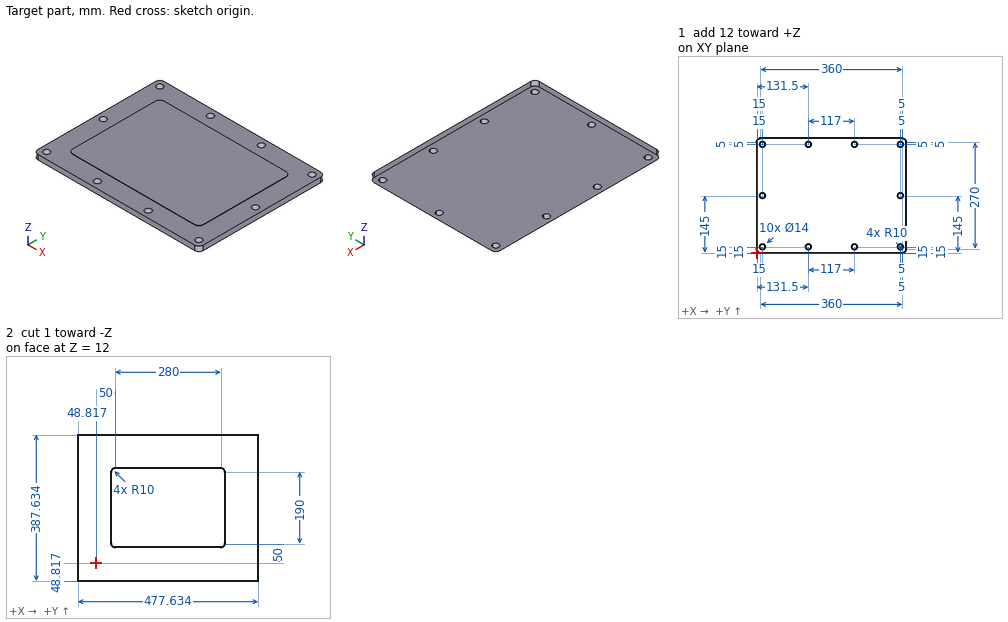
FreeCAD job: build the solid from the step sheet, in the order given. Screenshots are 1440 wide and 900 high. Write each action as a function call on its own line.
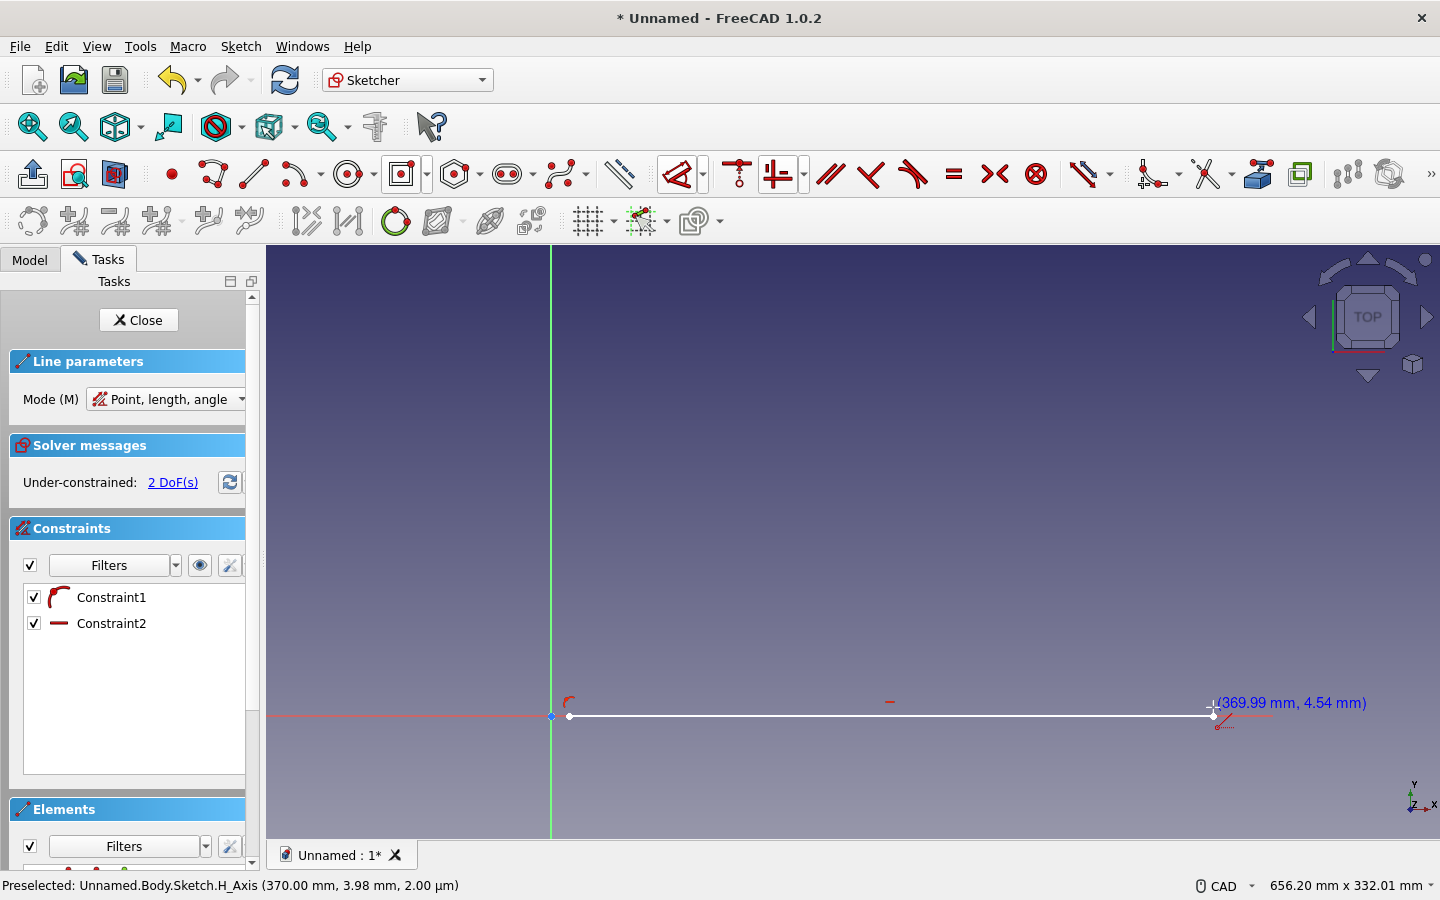
click(1231, 698)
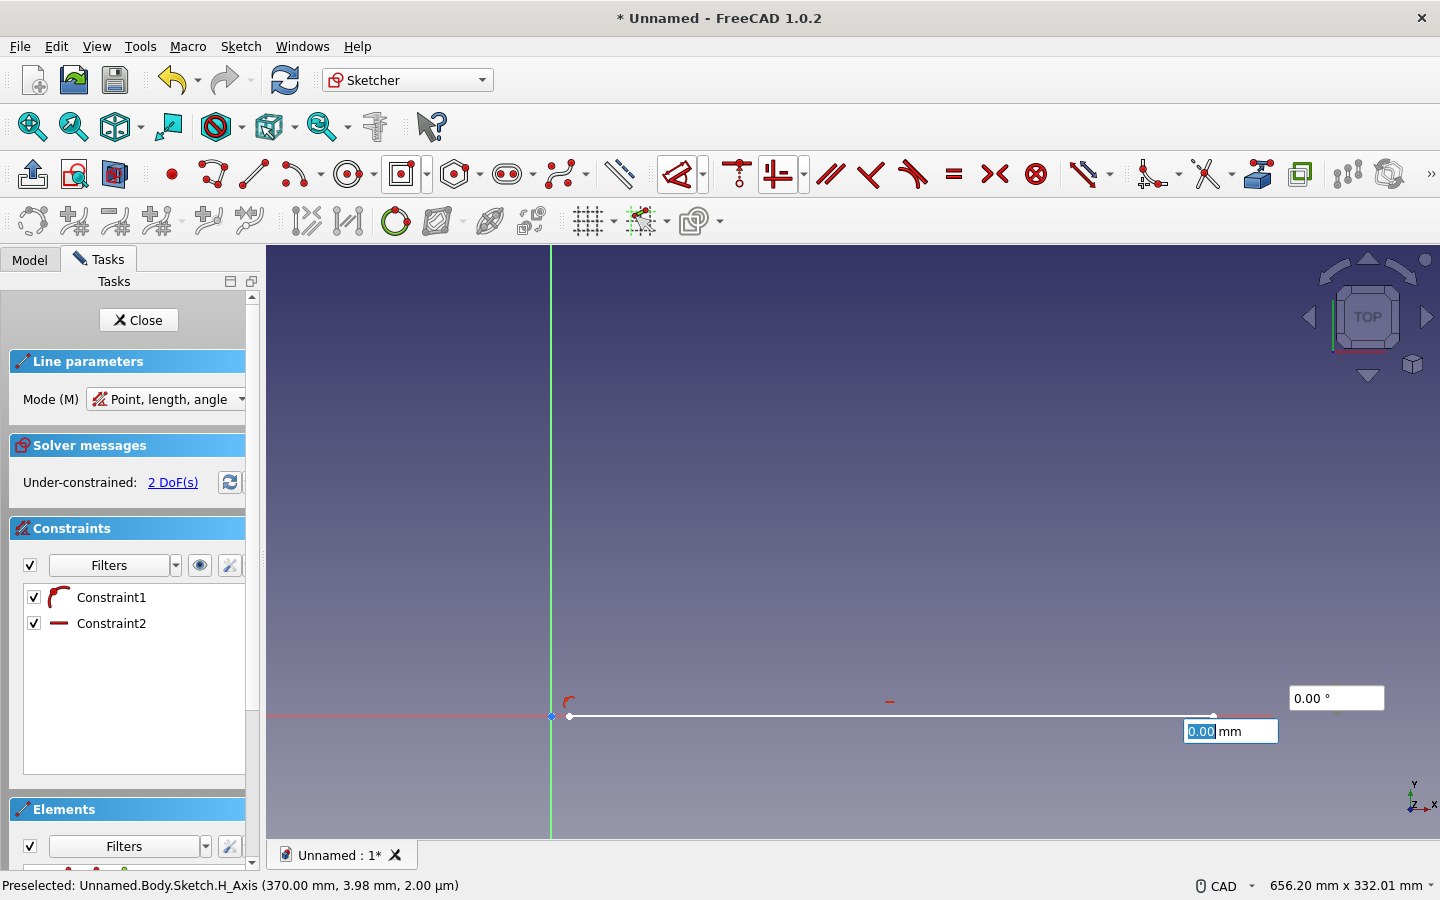
scroll(568, 715, down, 2)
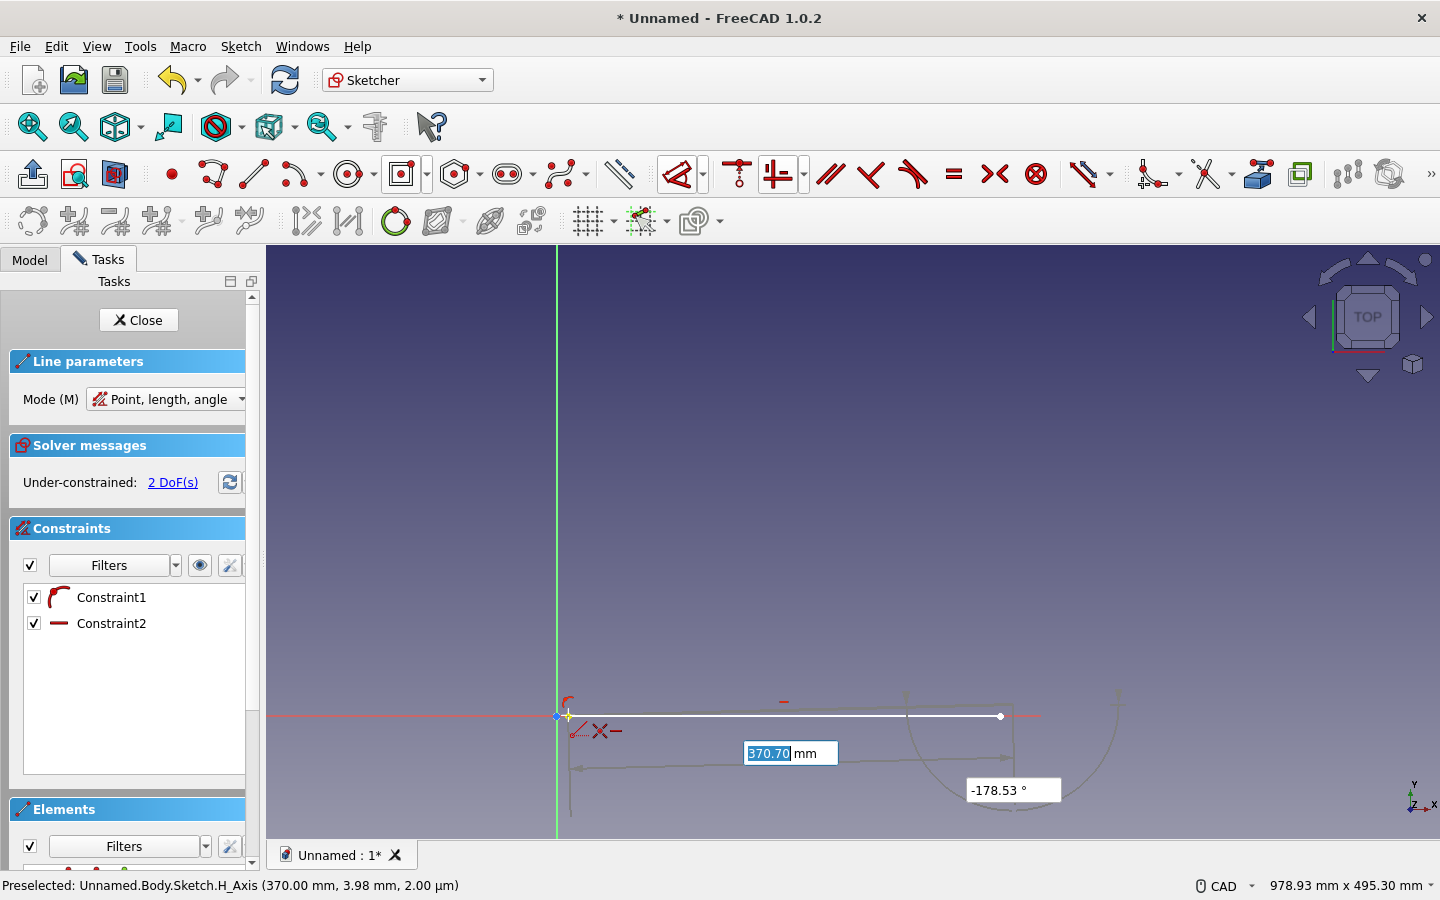
click(1013, 380)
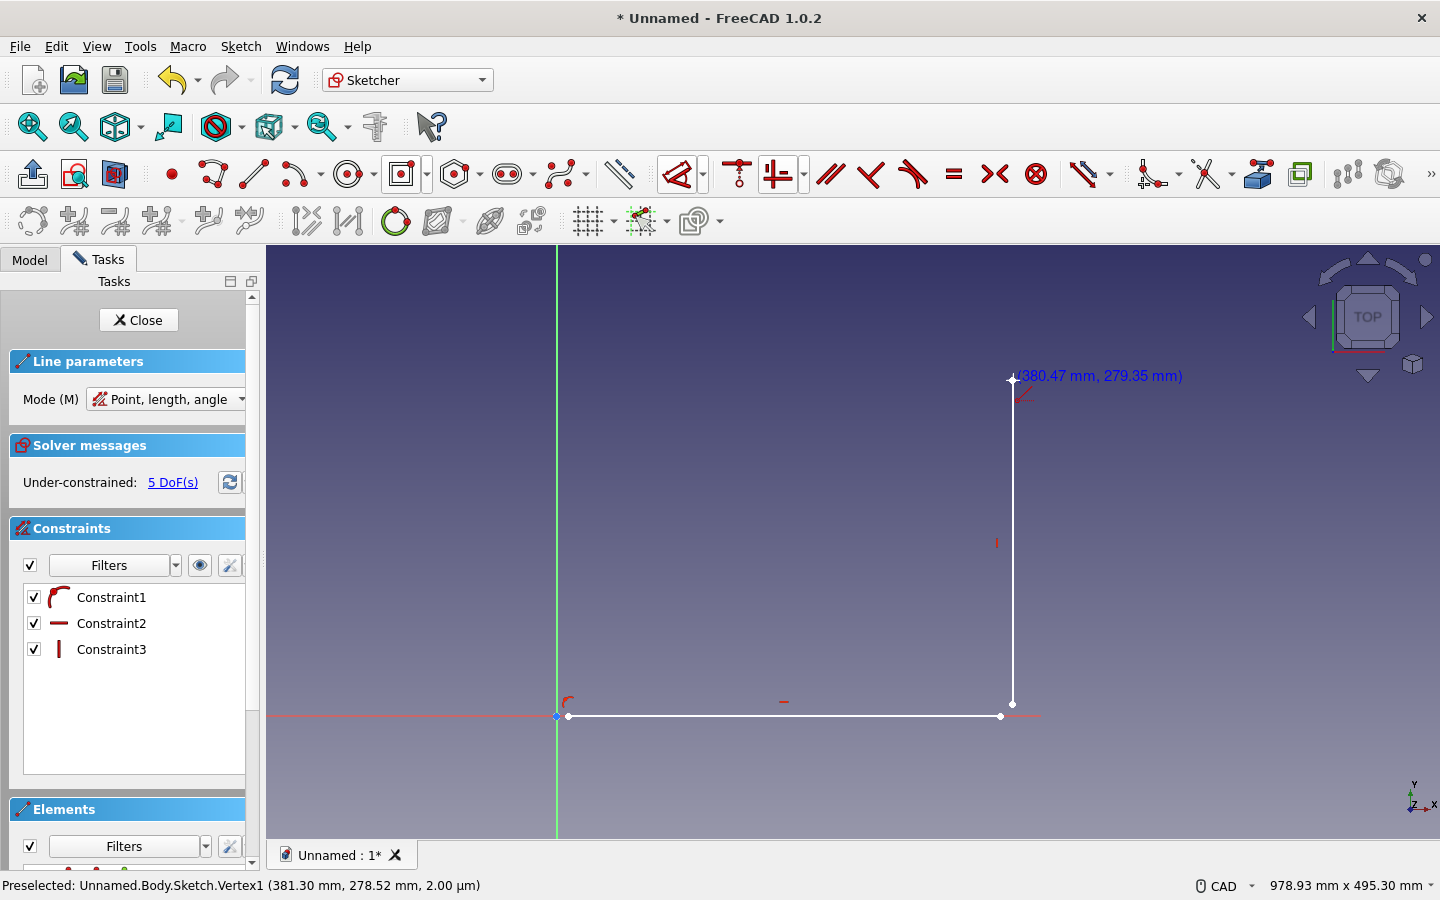
click(1000, 368)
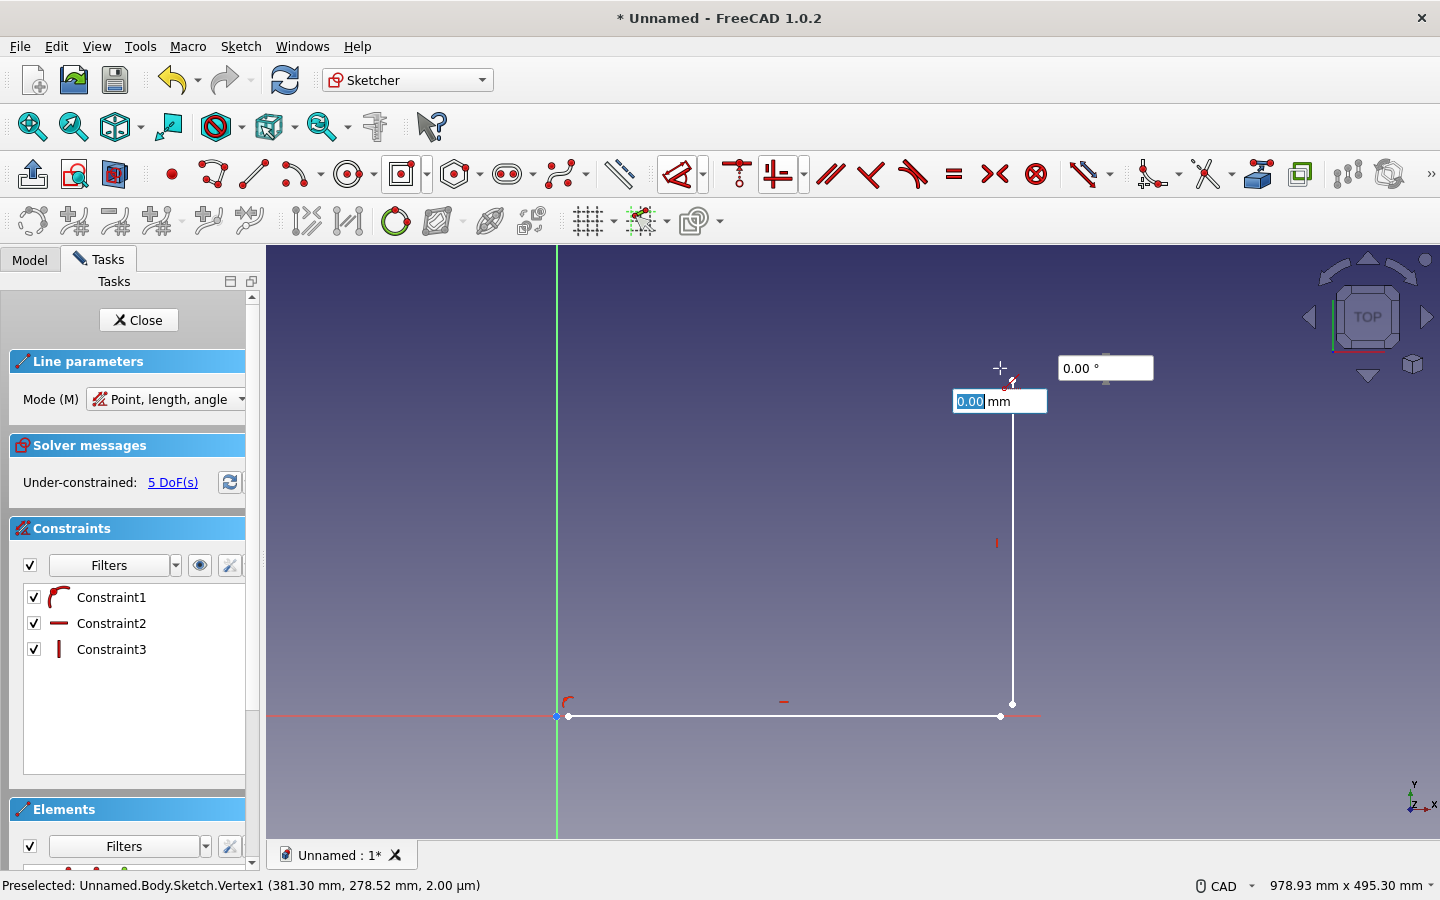
scroll(569, 368, up, 2)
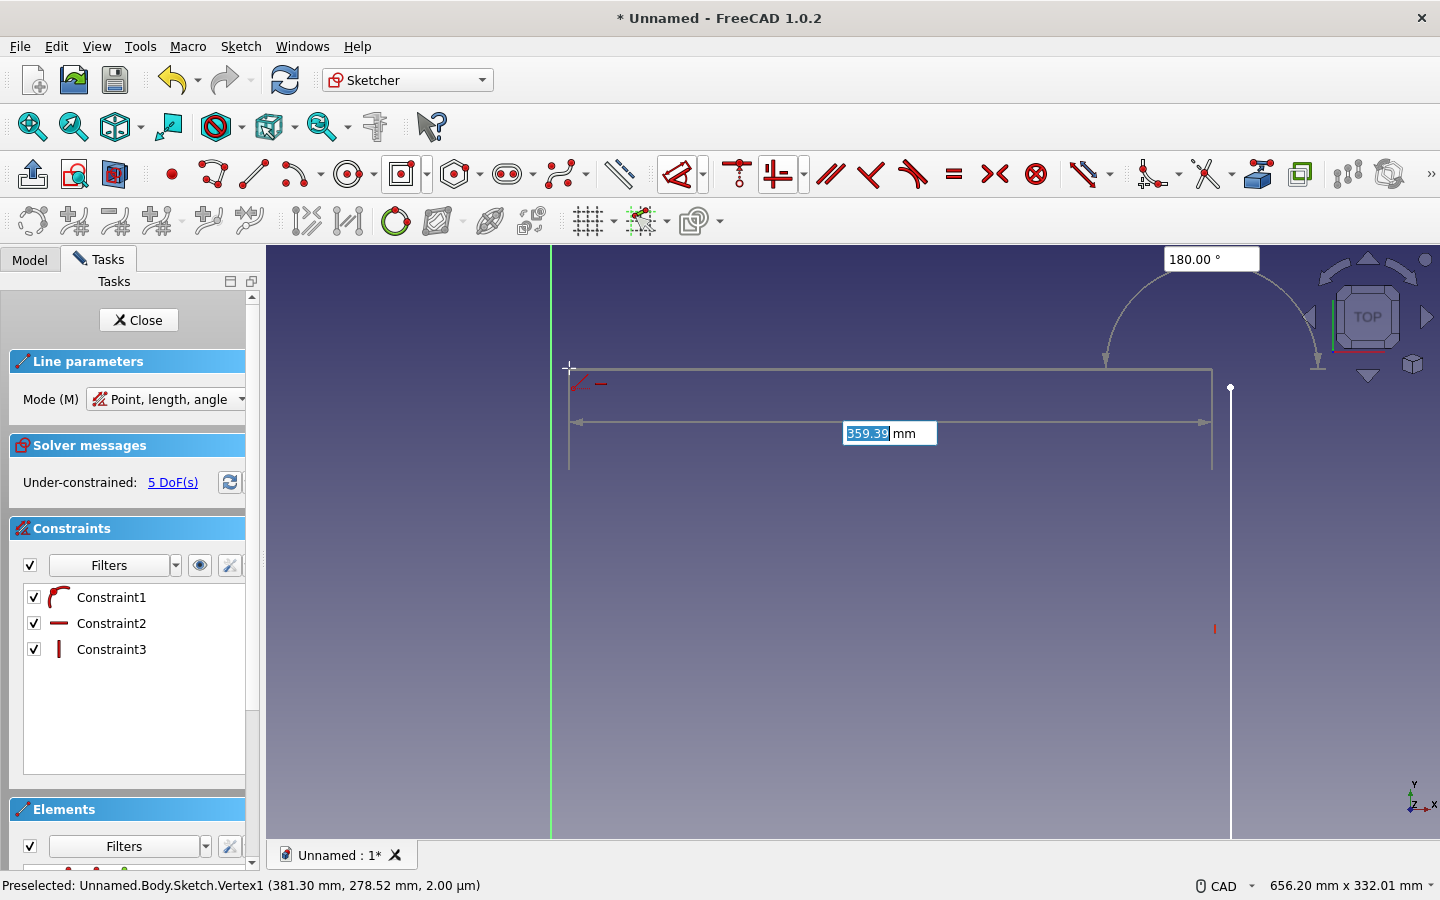
click(568, 368)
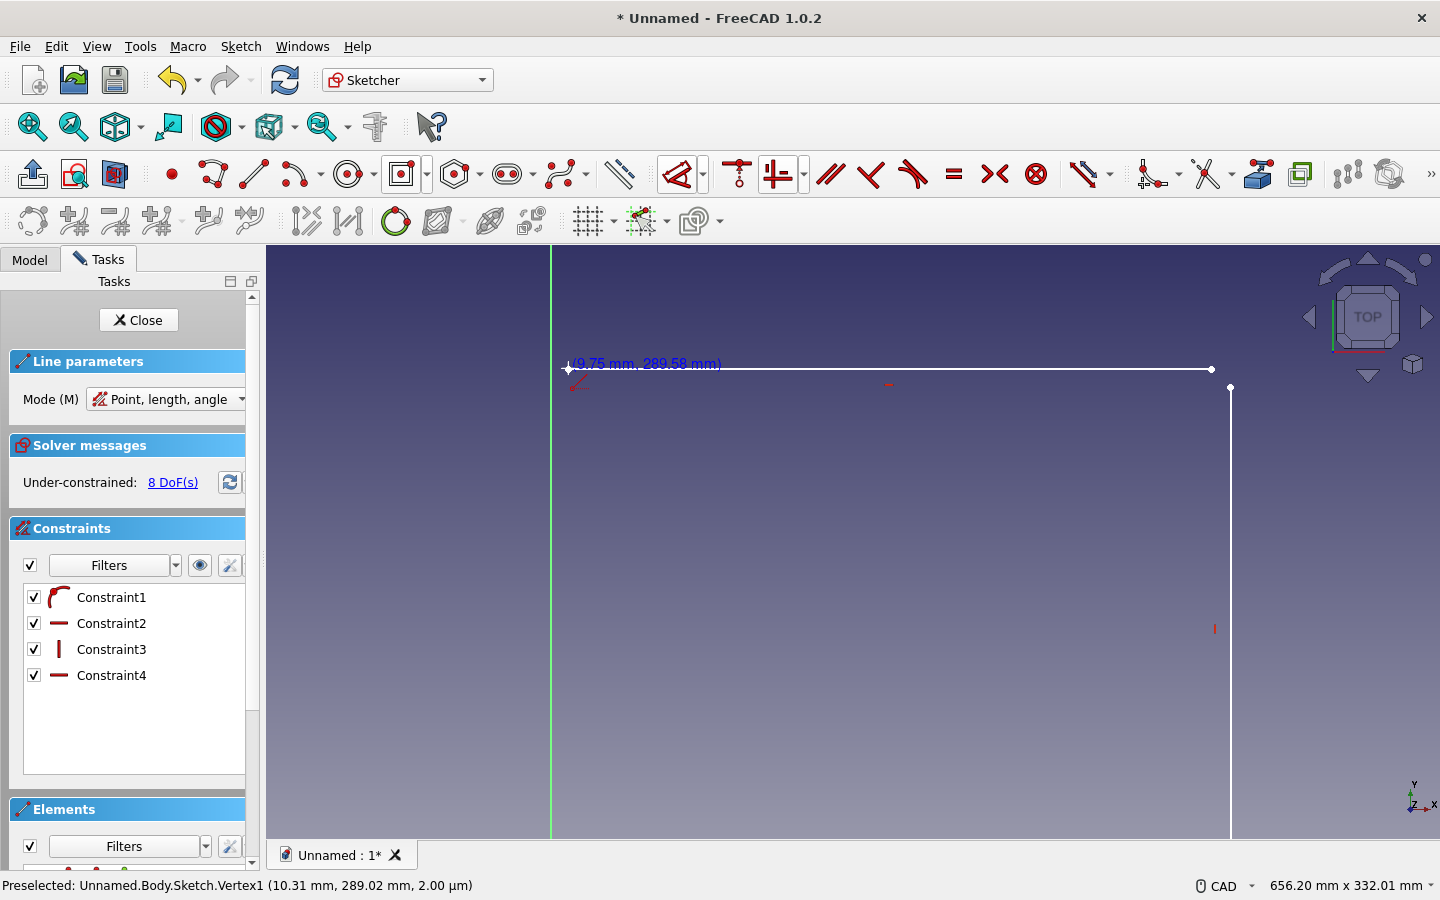
click(551, 386)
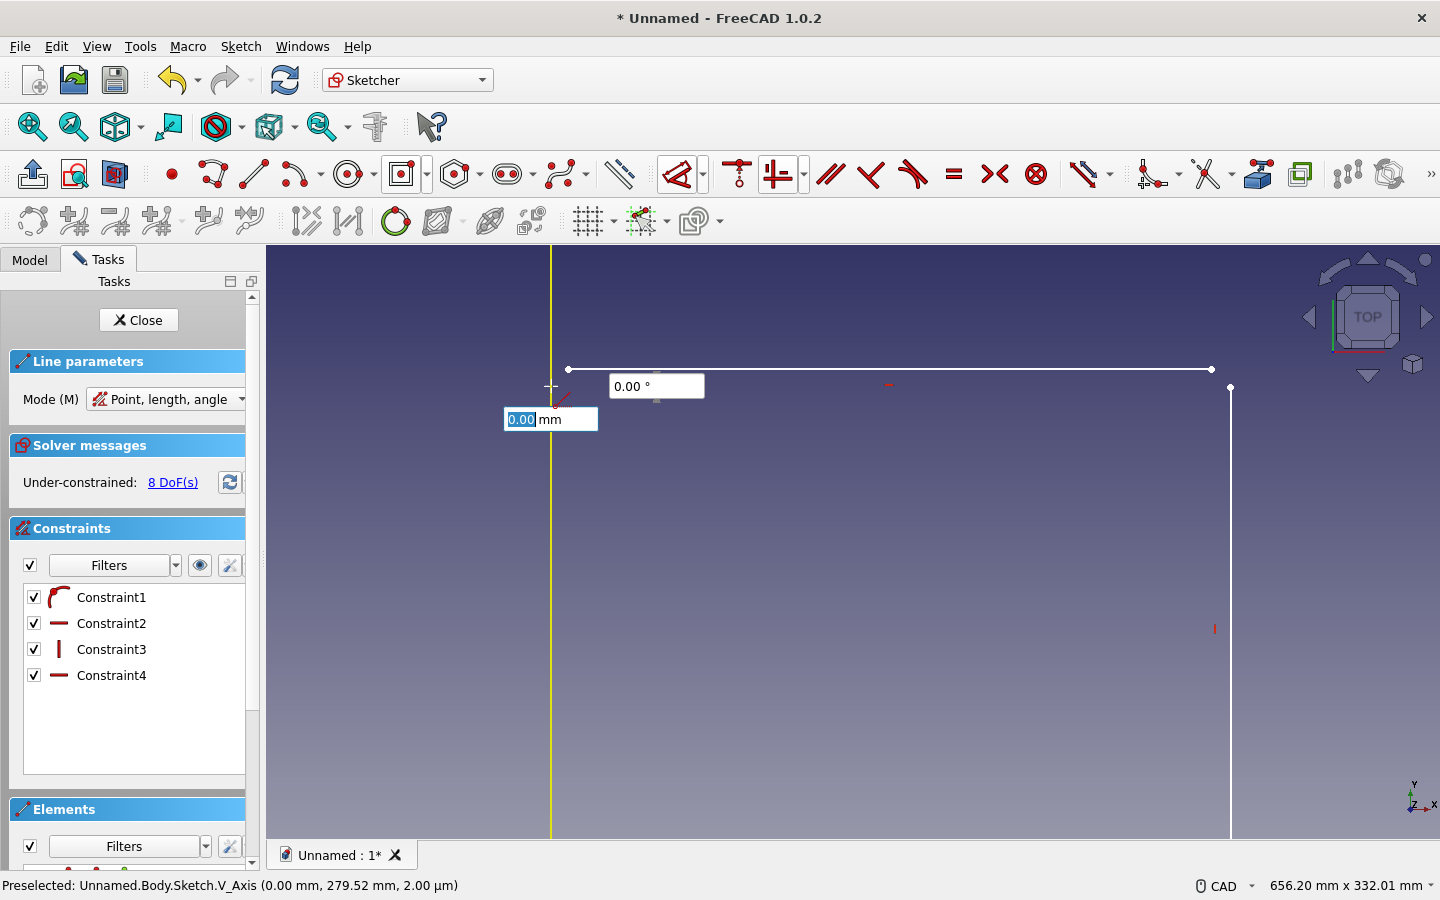
scroll(569, 368, down, 2)